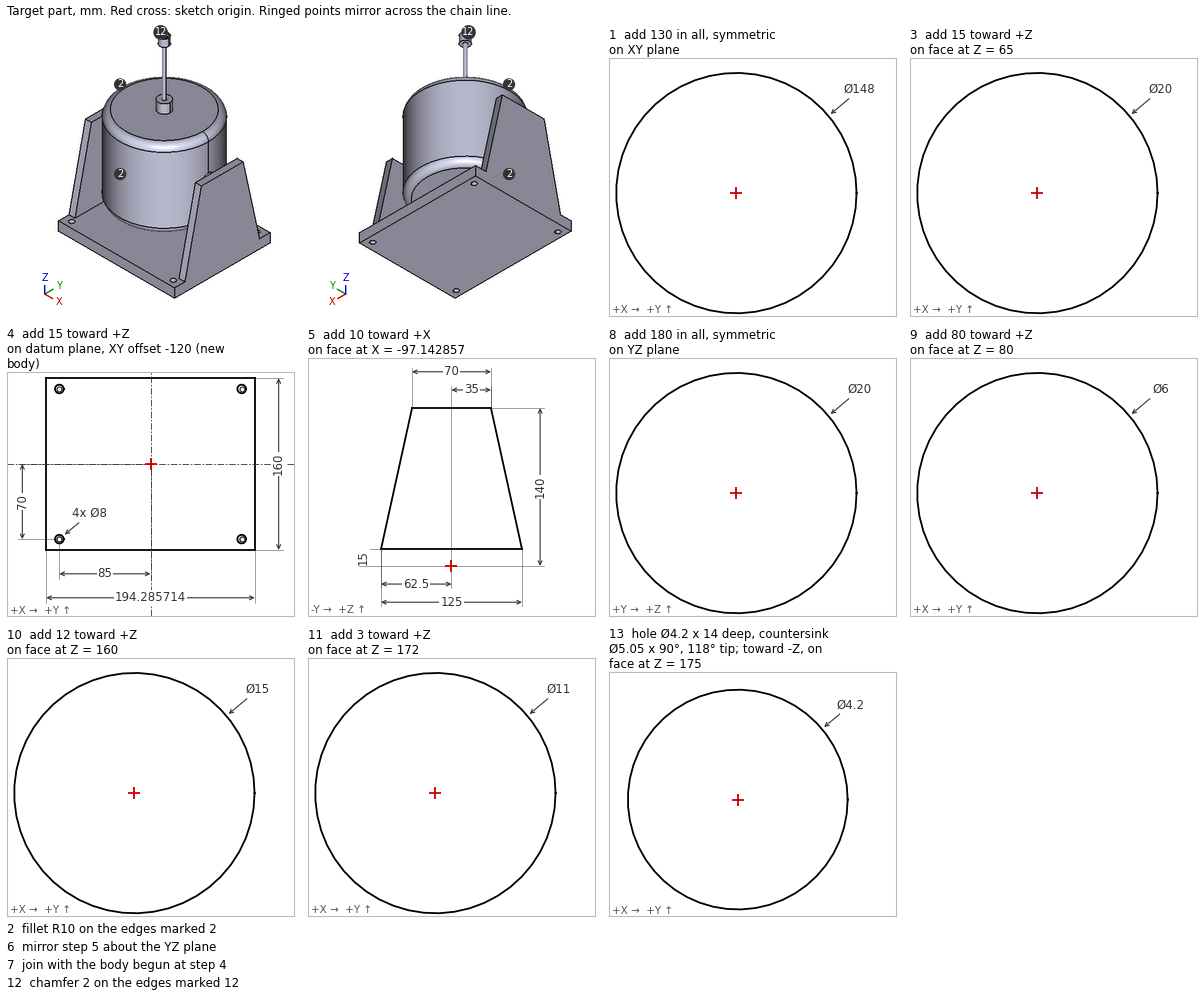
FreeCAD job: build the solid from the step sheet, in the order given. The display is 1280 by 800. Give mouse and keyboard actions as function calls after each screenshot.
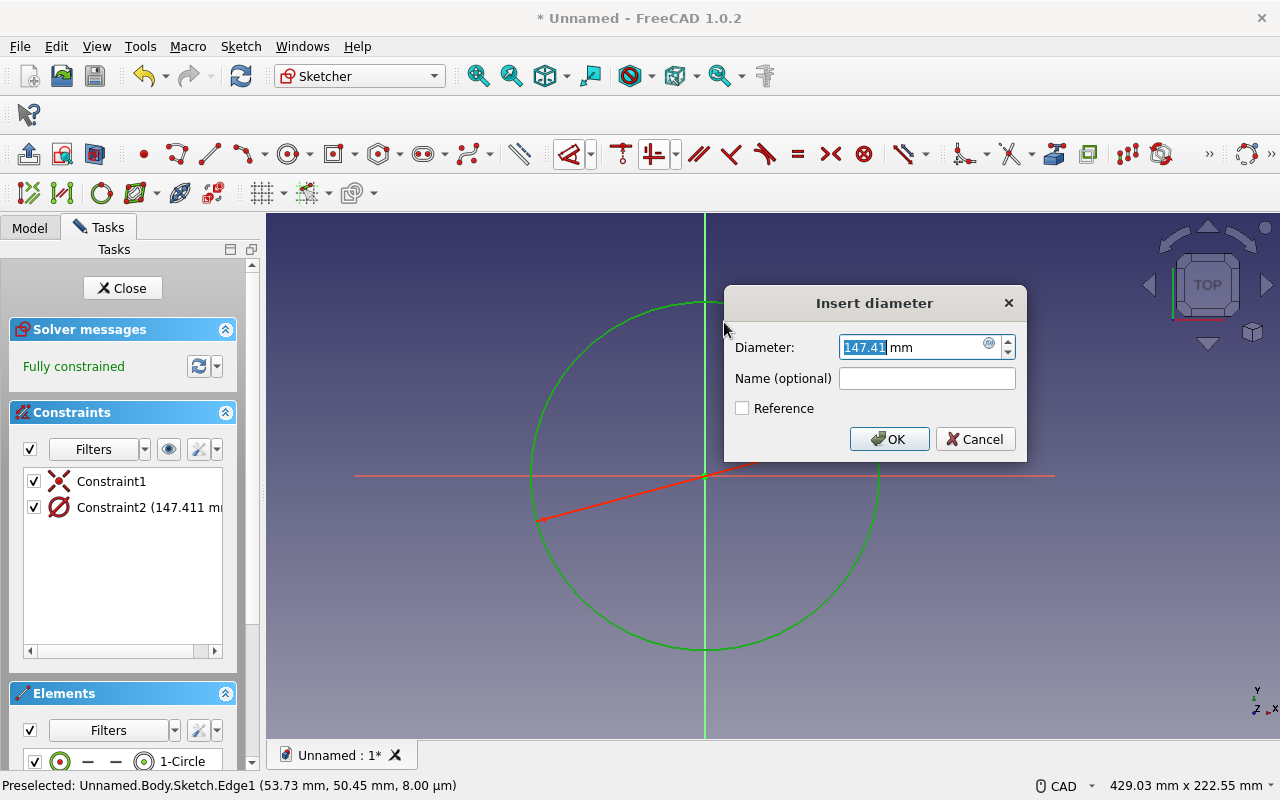
text(148)
key(Return)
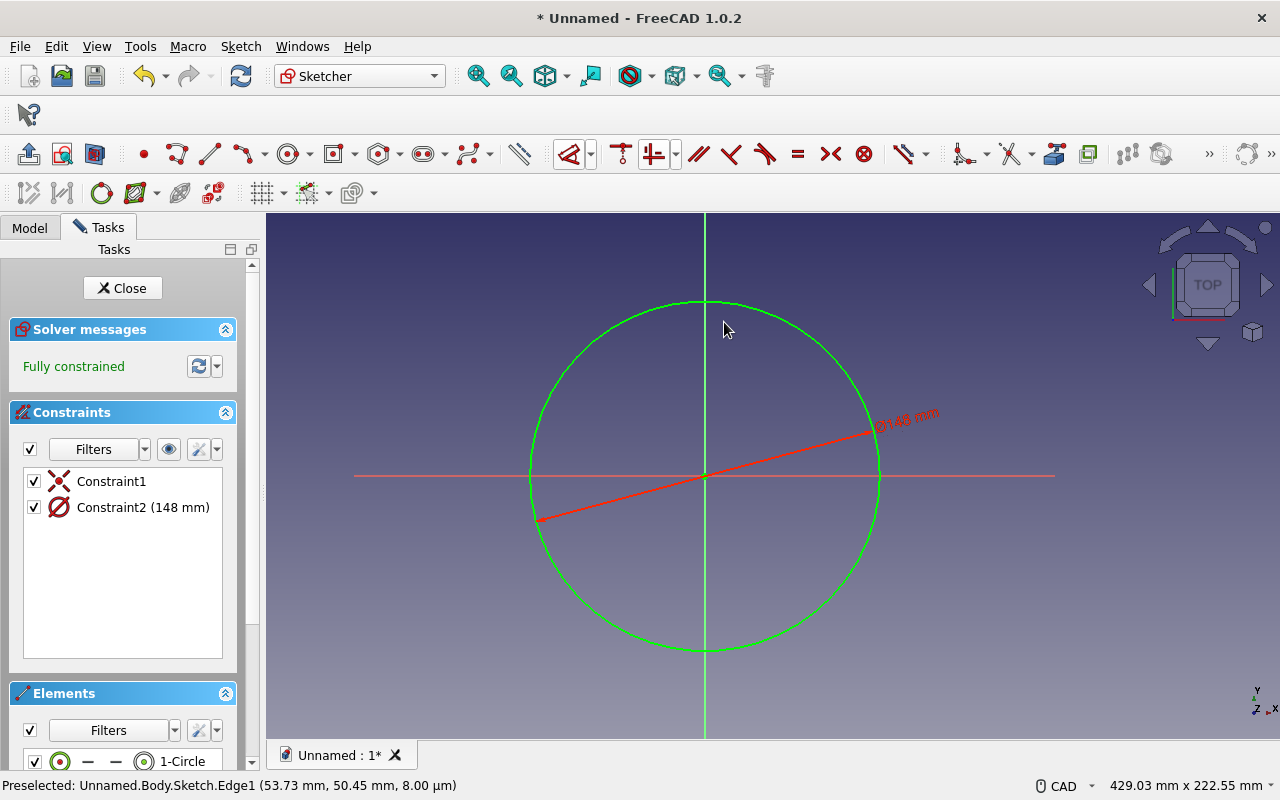
click(123, 288)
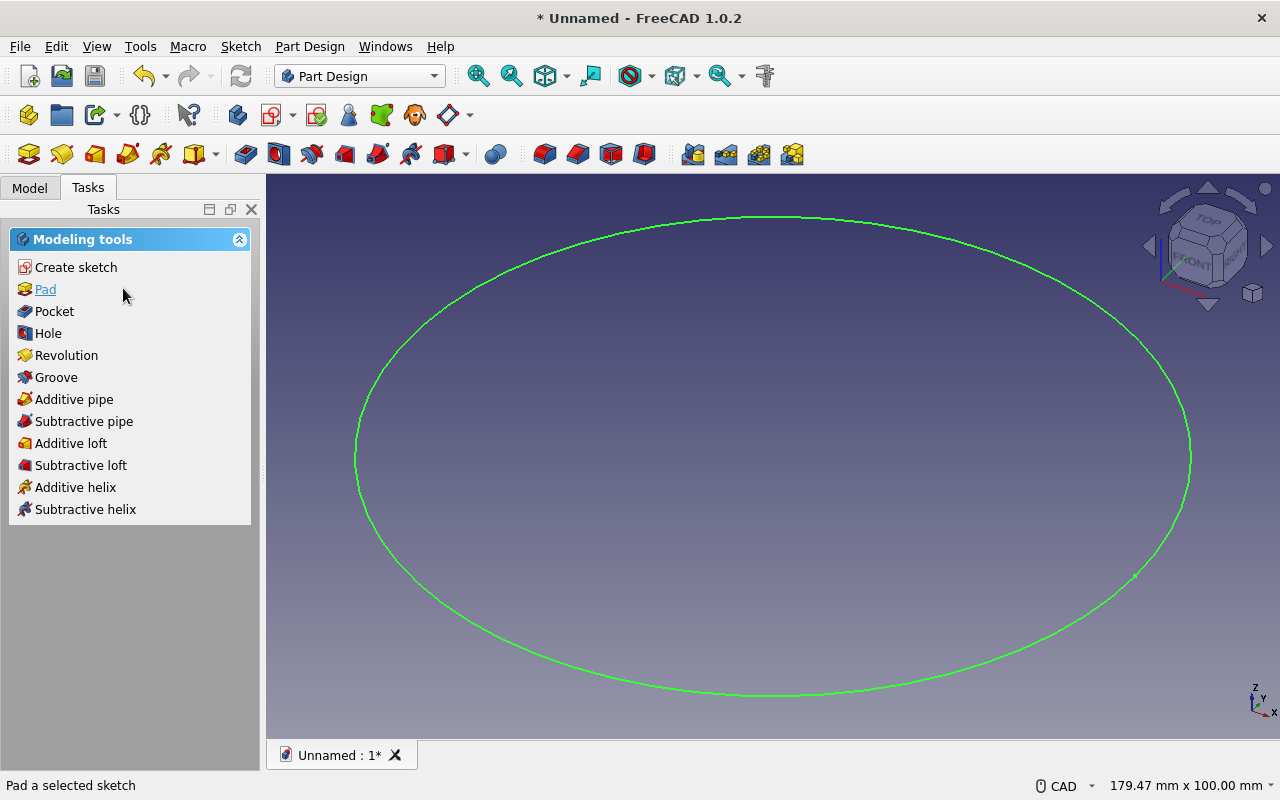
click(29, 154)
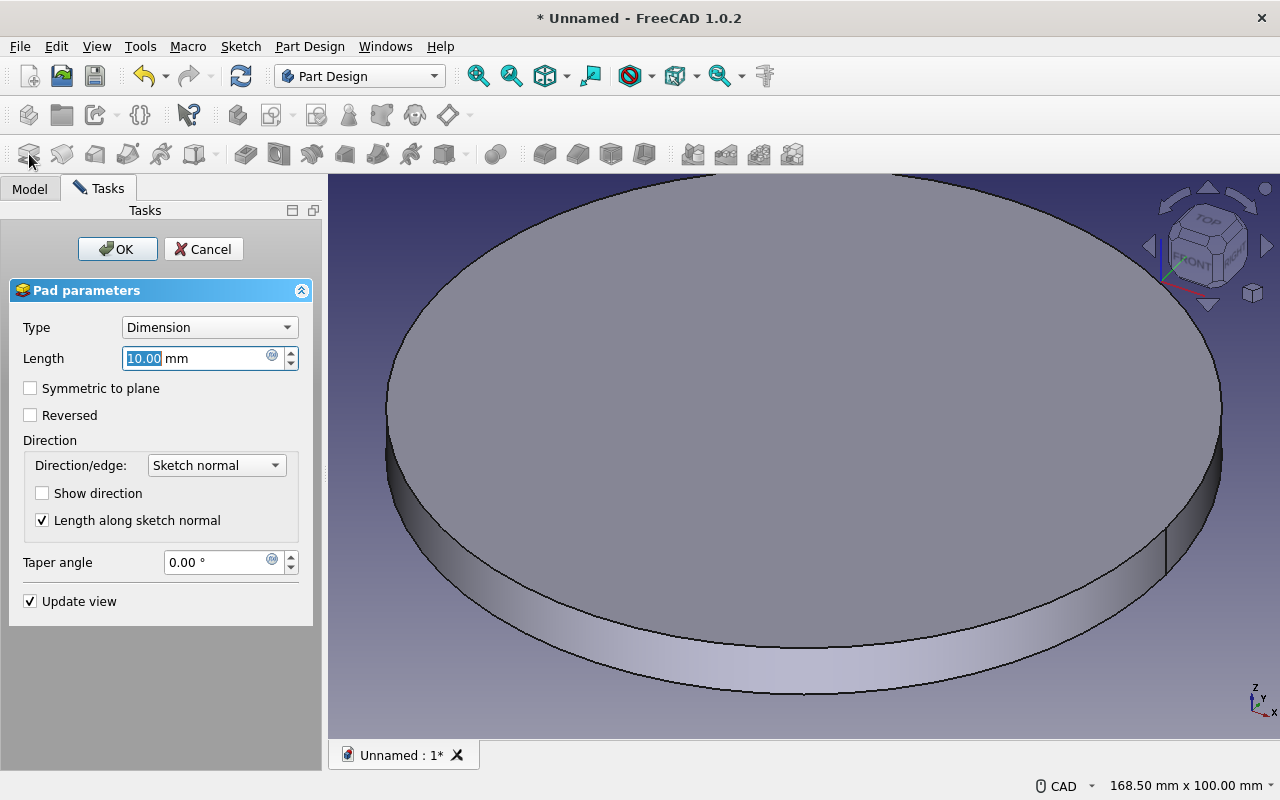
text(130)
key(Tab)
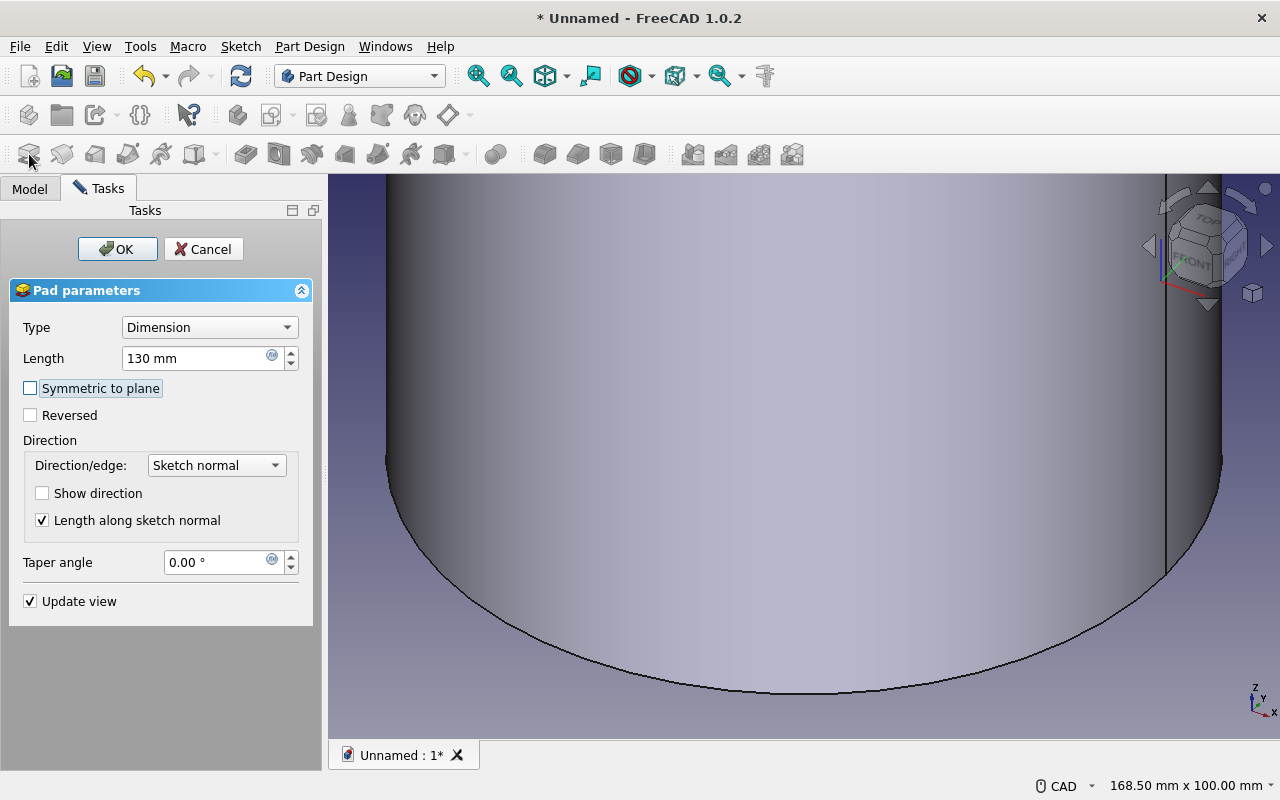
click(31, 388)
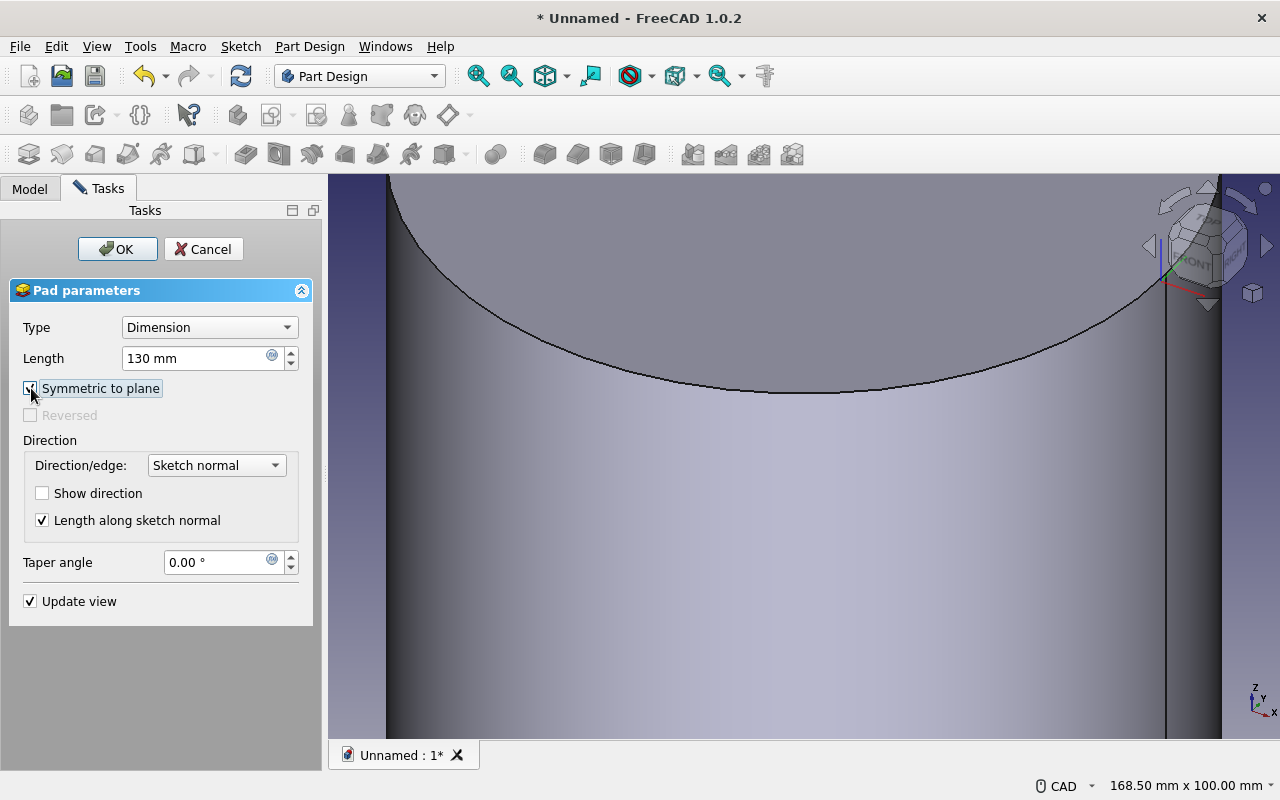
click(118, 249)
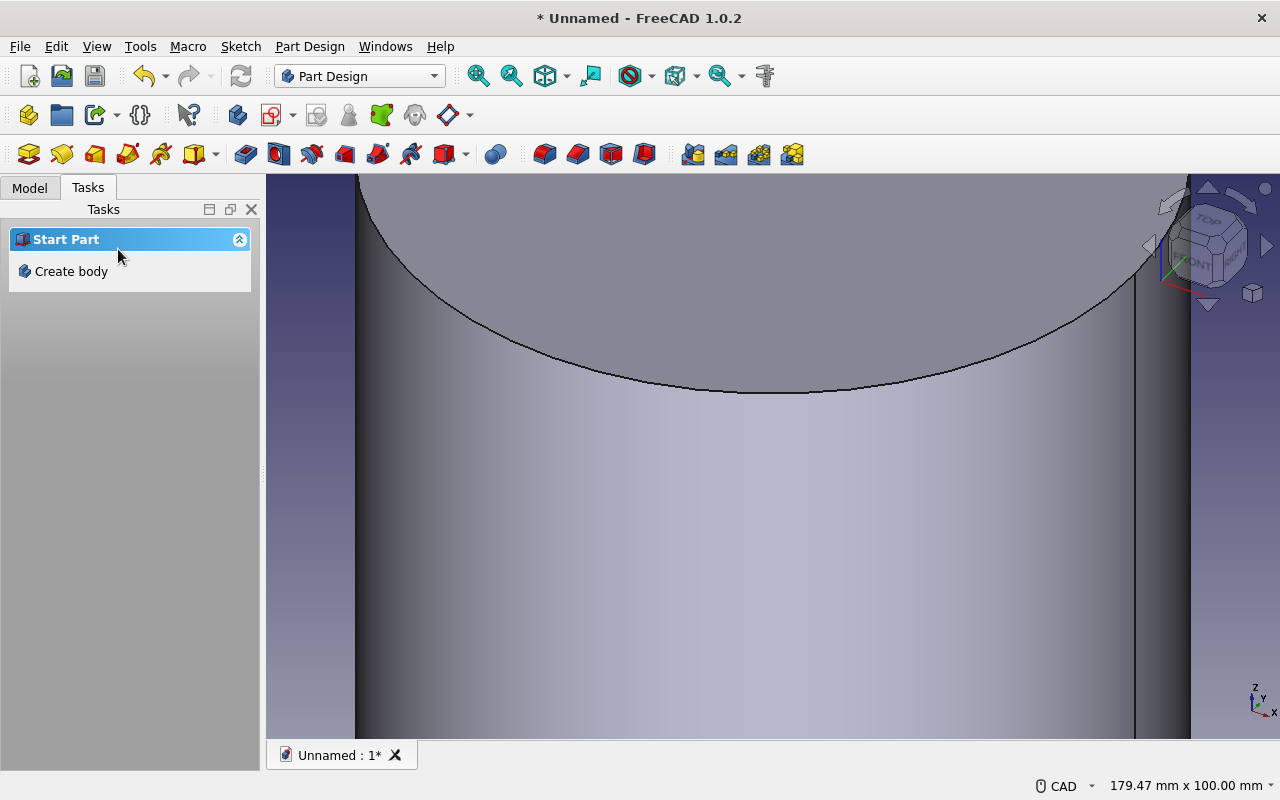
key(v)
key(f)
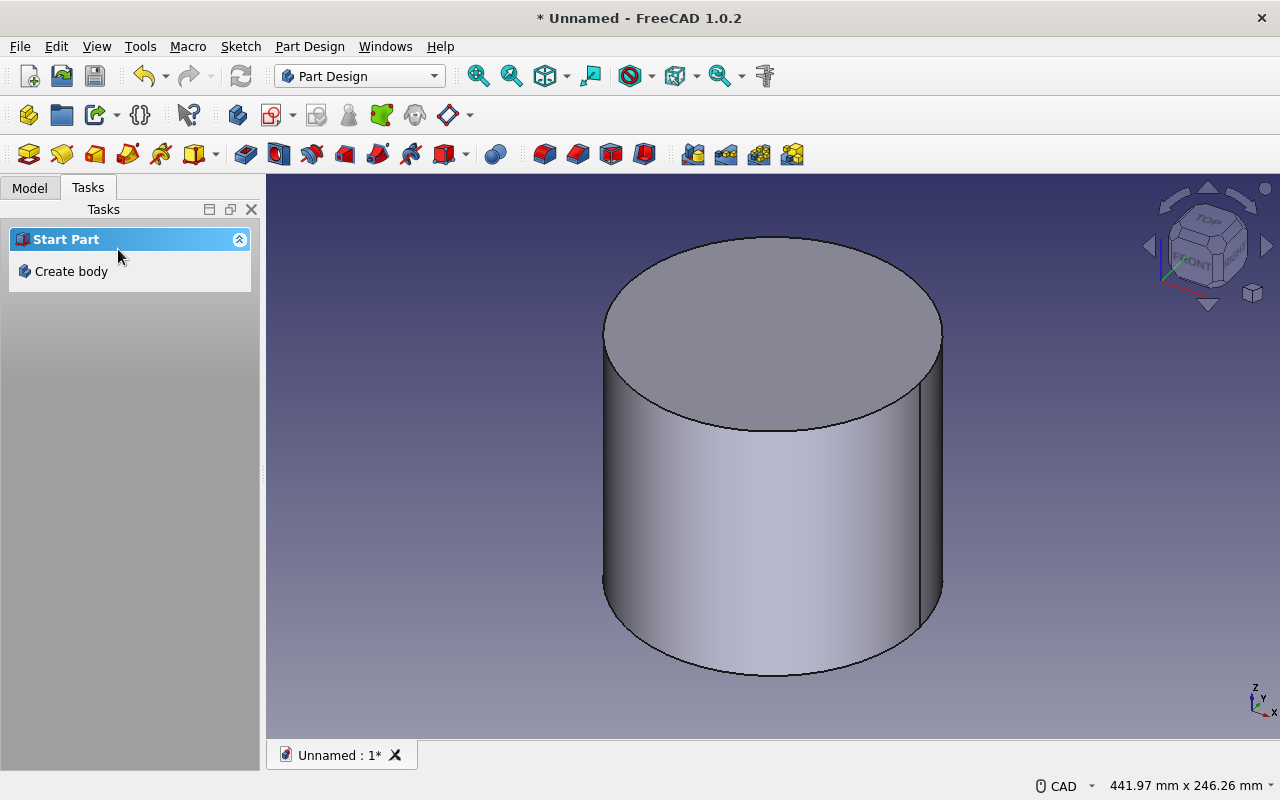
click(604, 343)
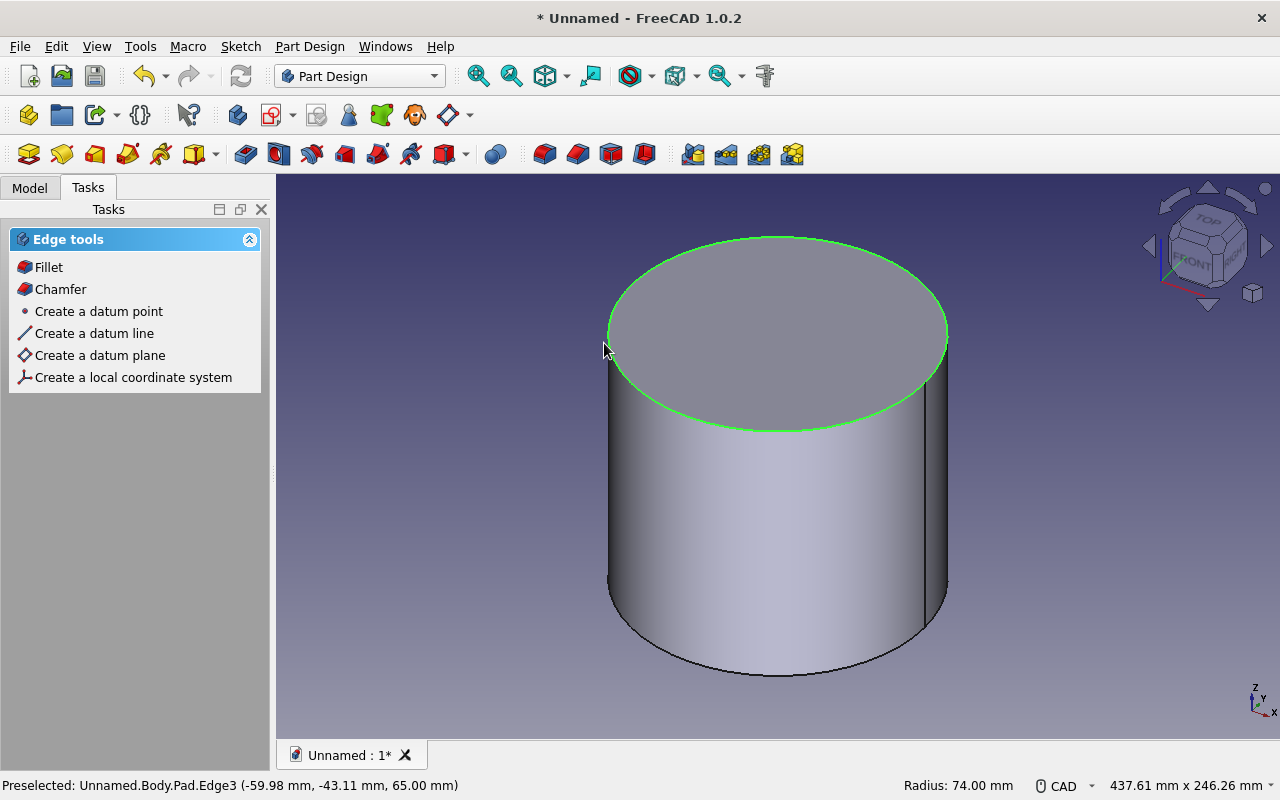
key(0)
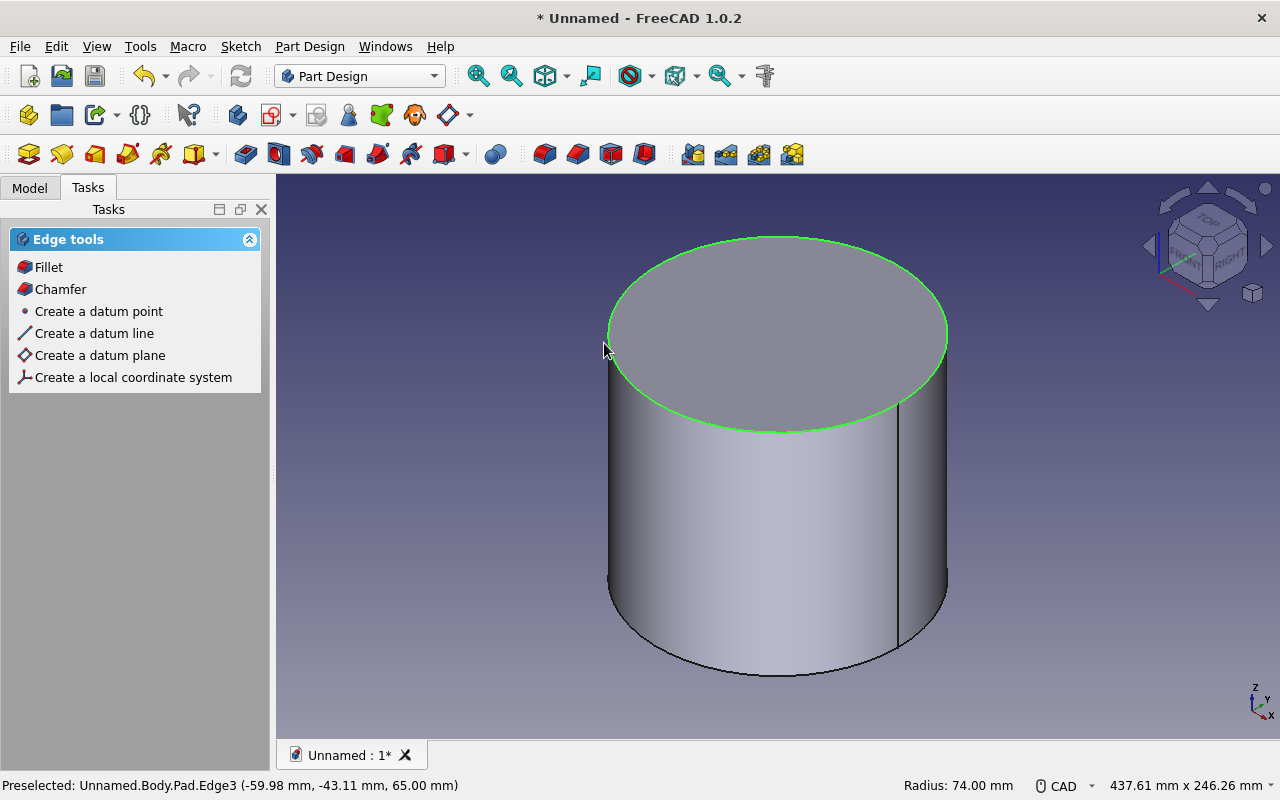
key(2)